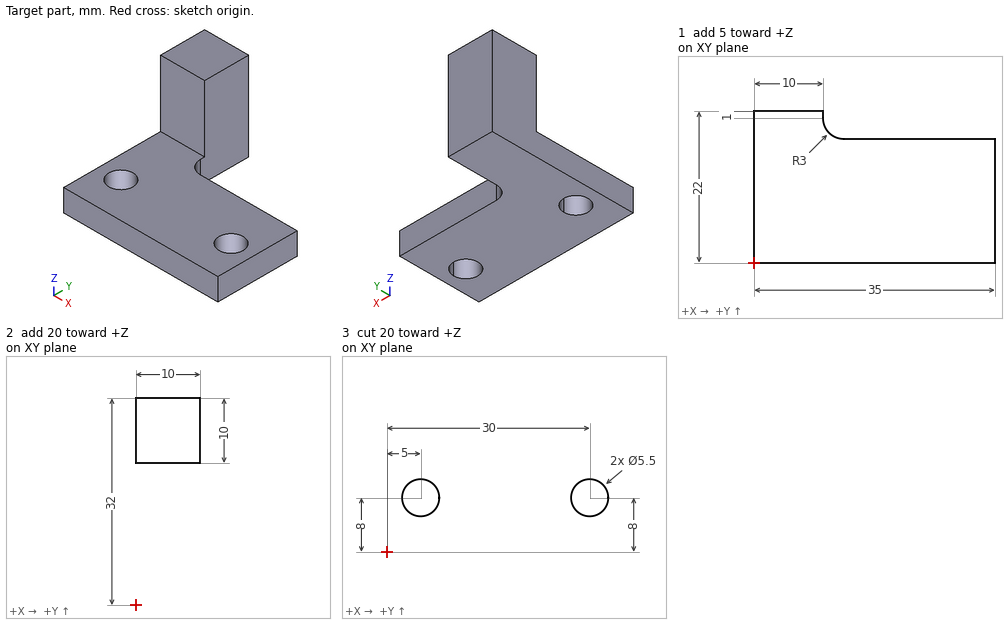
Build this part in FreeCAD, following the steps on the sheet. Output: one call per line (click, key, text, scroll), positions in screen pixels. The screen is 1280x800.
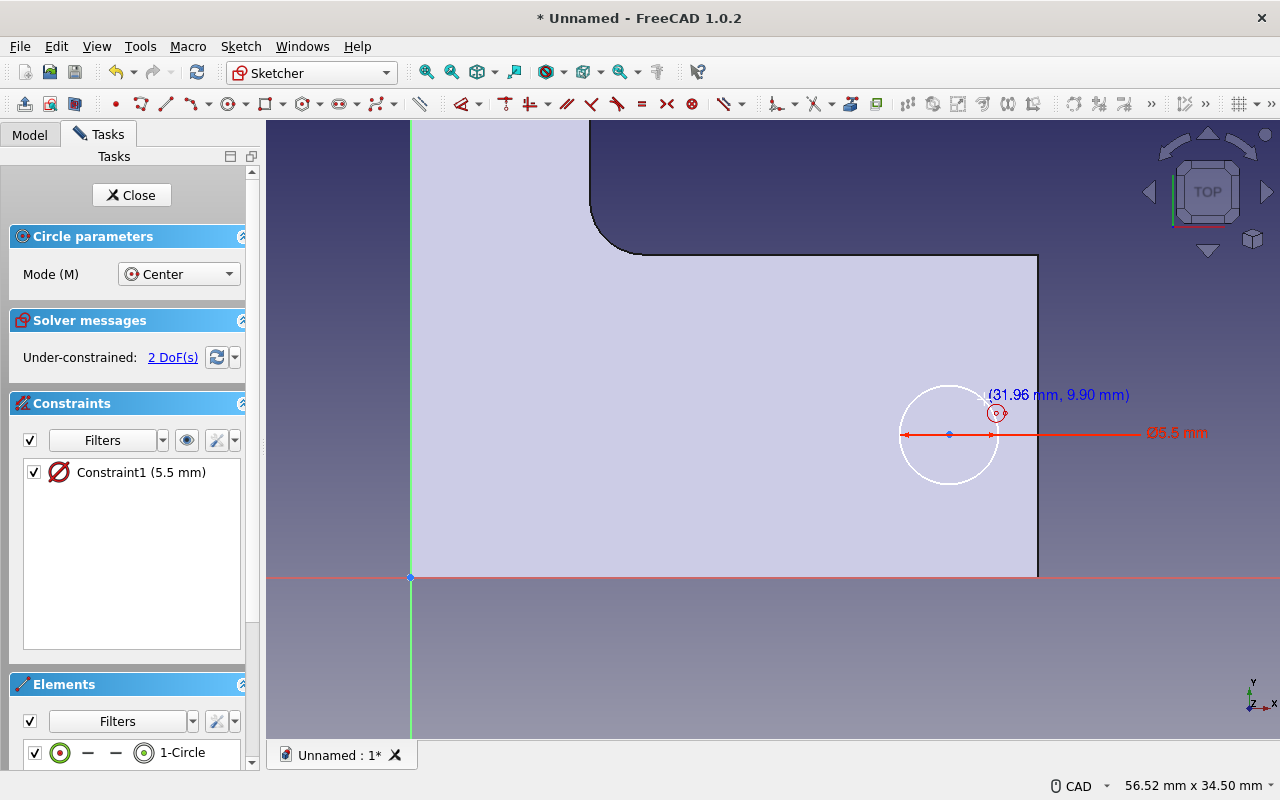
click(500, 434)
move(535, 399)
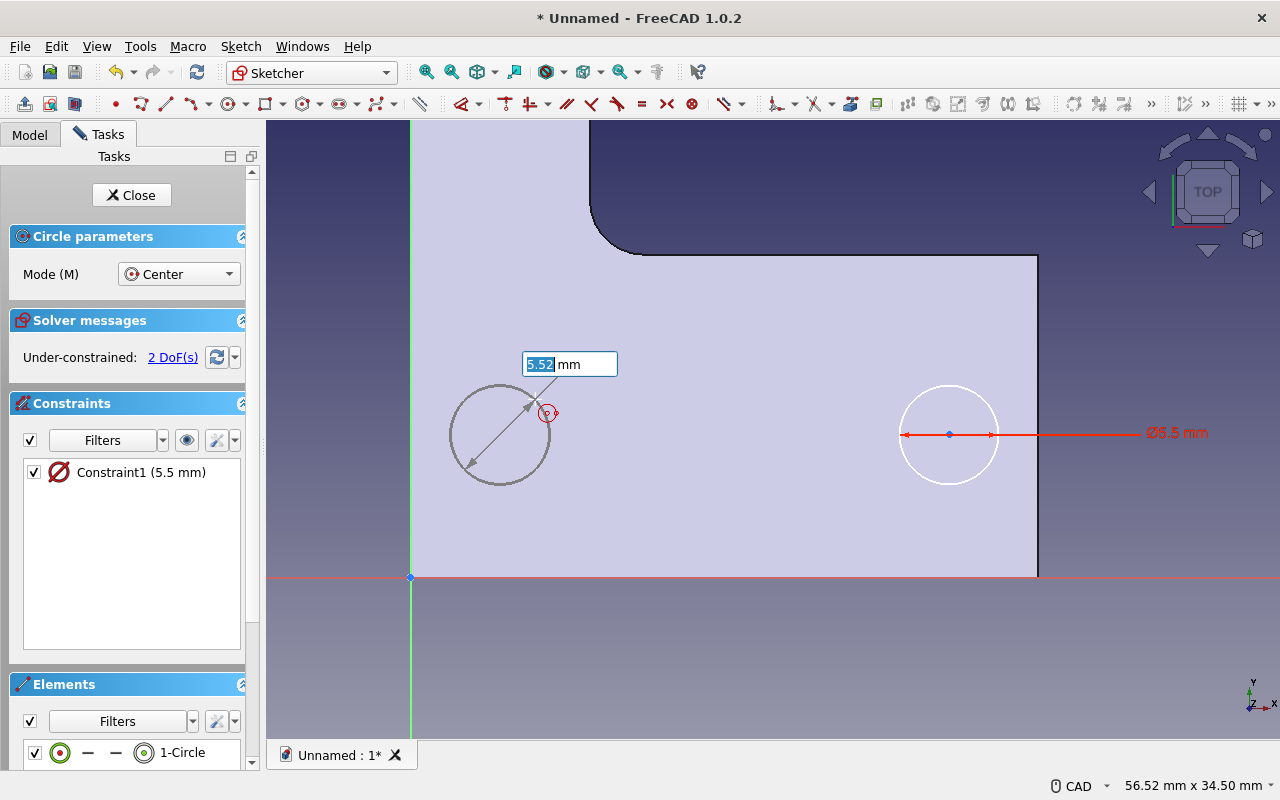
text(5.5)
key(Return)
key(Escape)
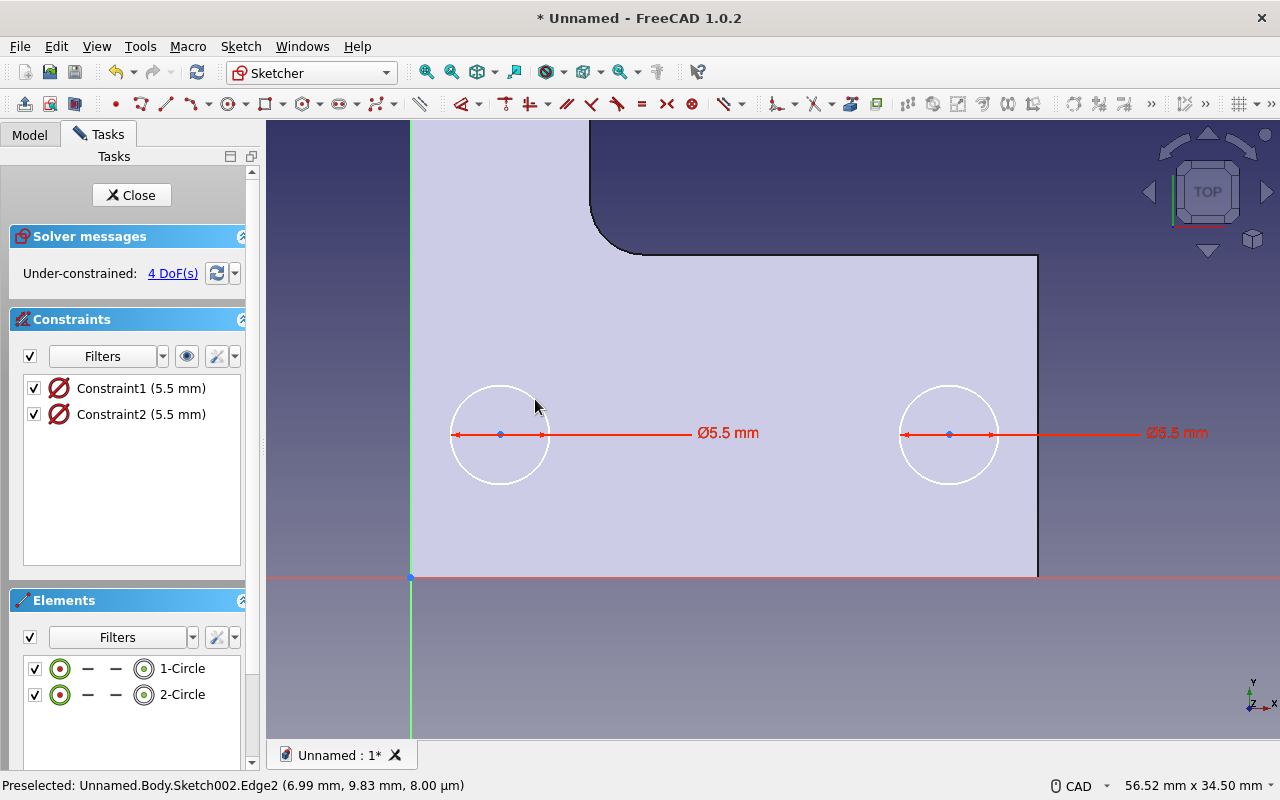
key(d)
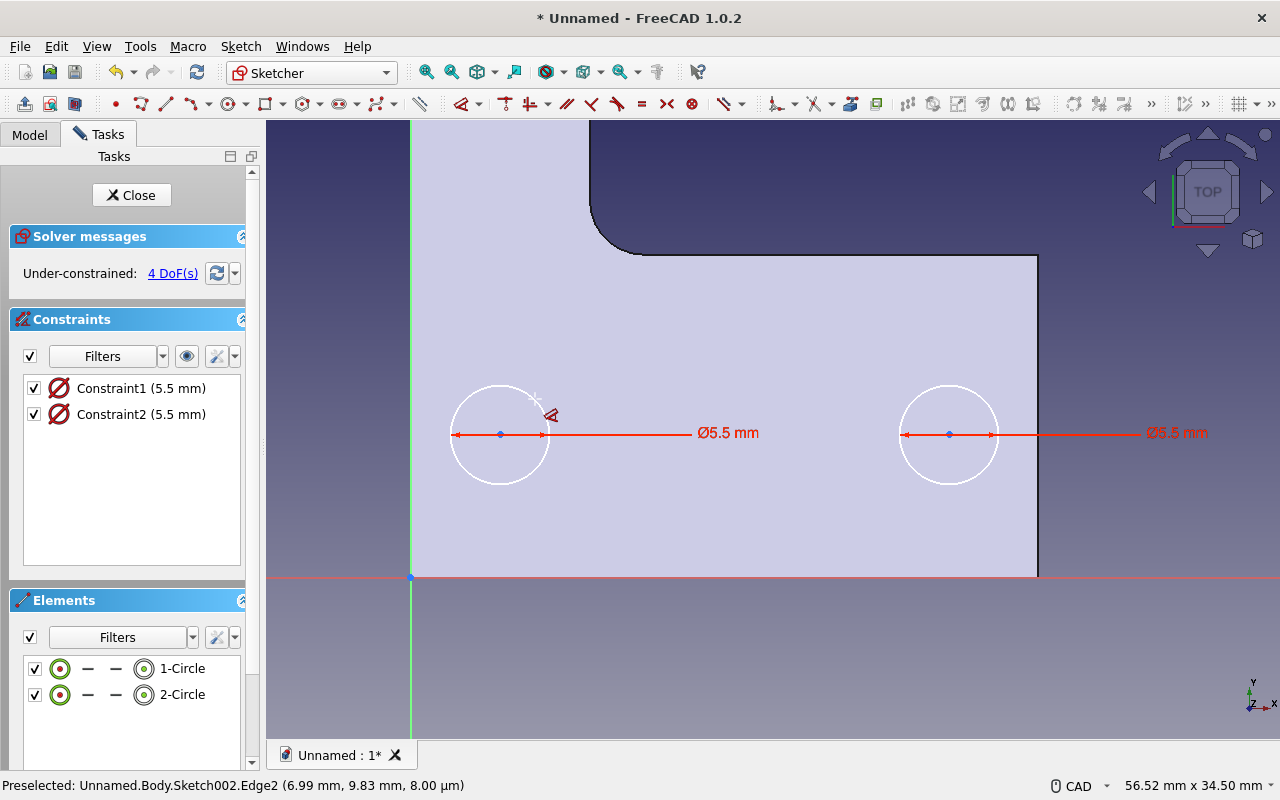
click(949, 435)
click(377, 506)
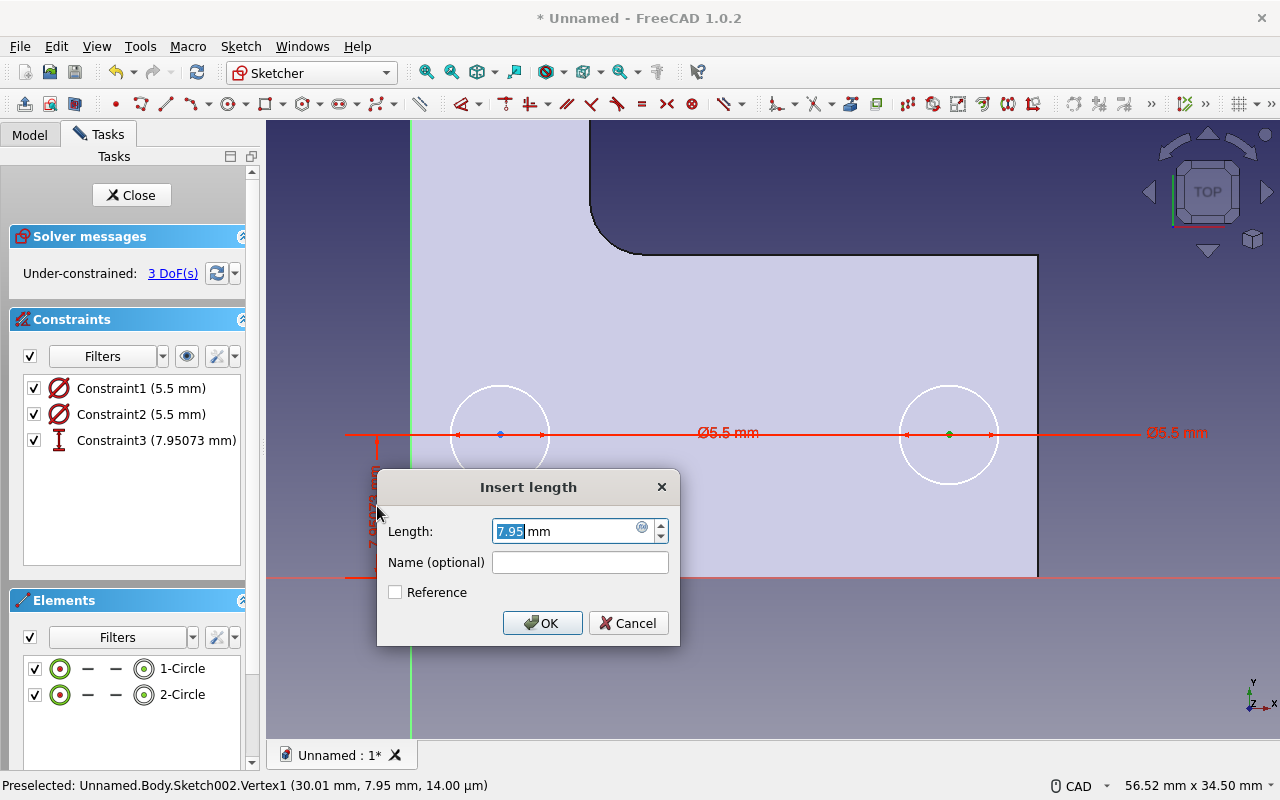
text(8)
key(Return)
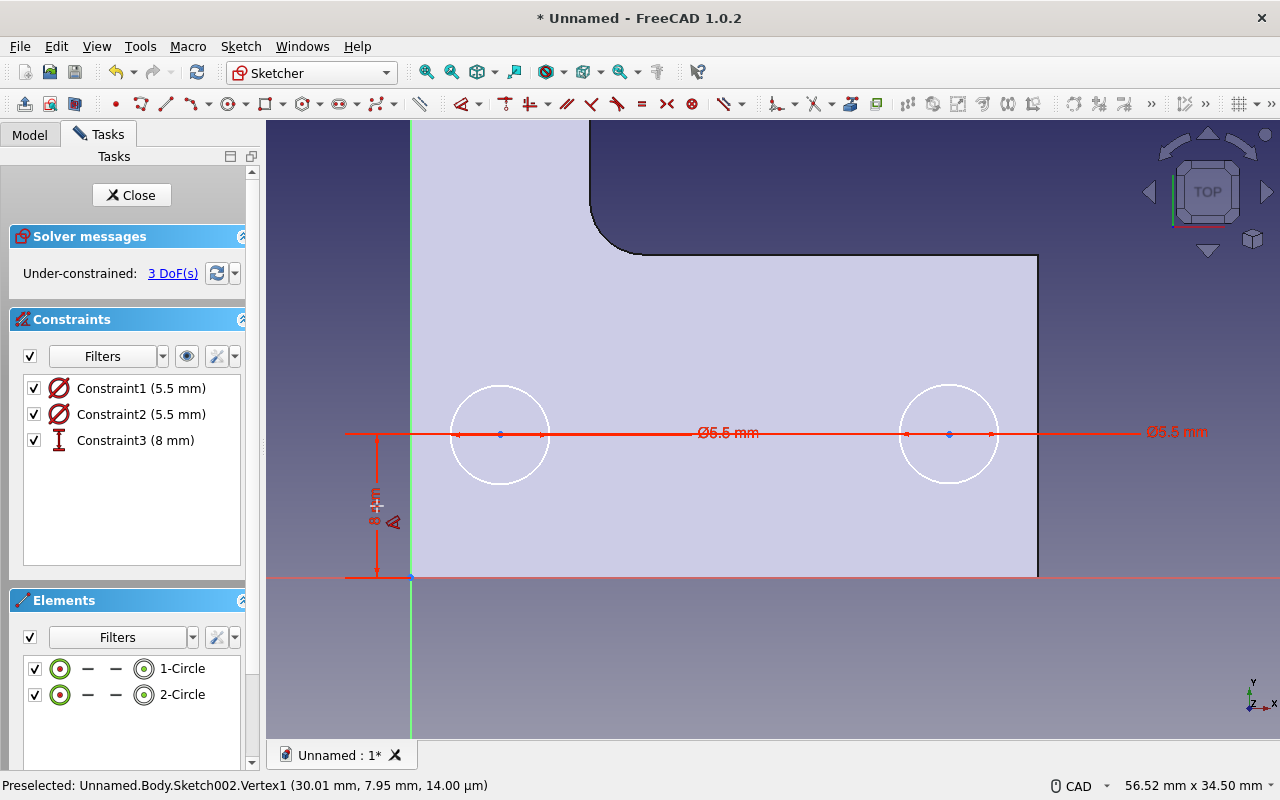
click(500, 435)
click(455, 612)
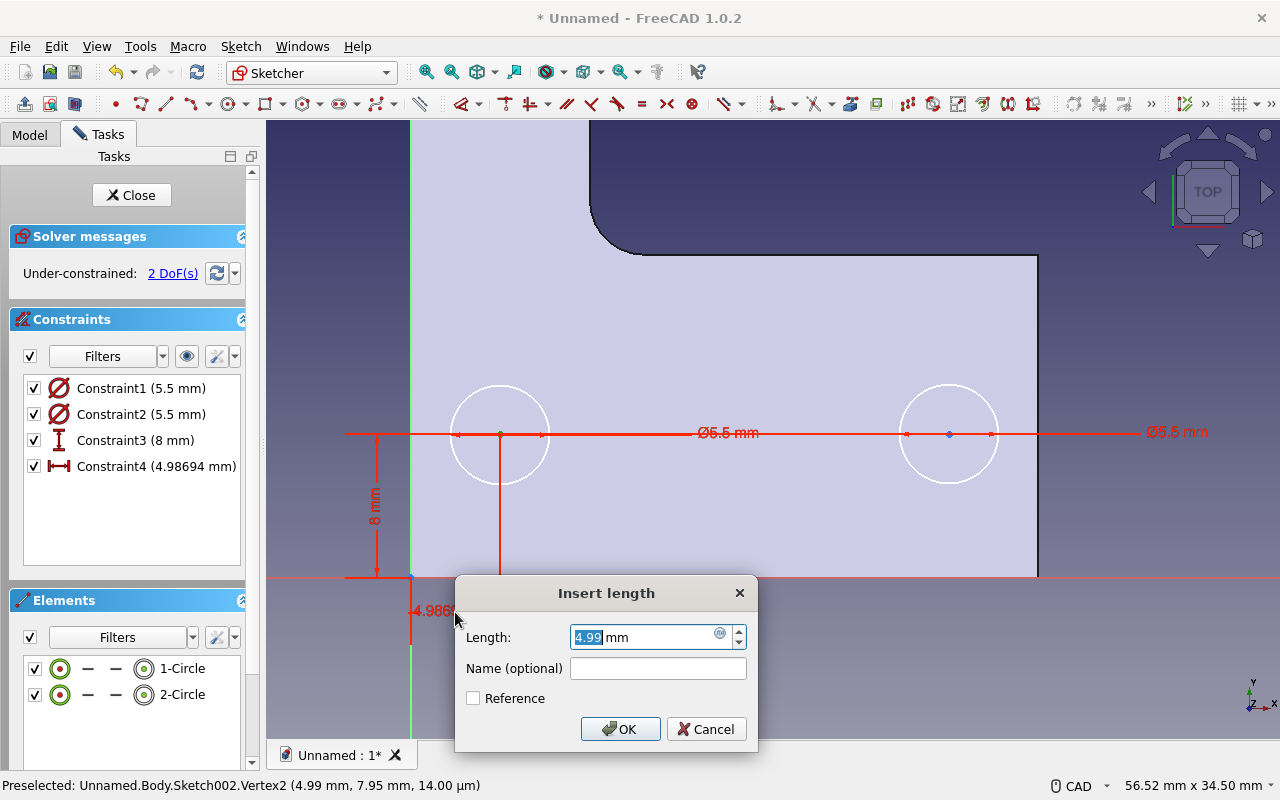
text(5)
key(Return)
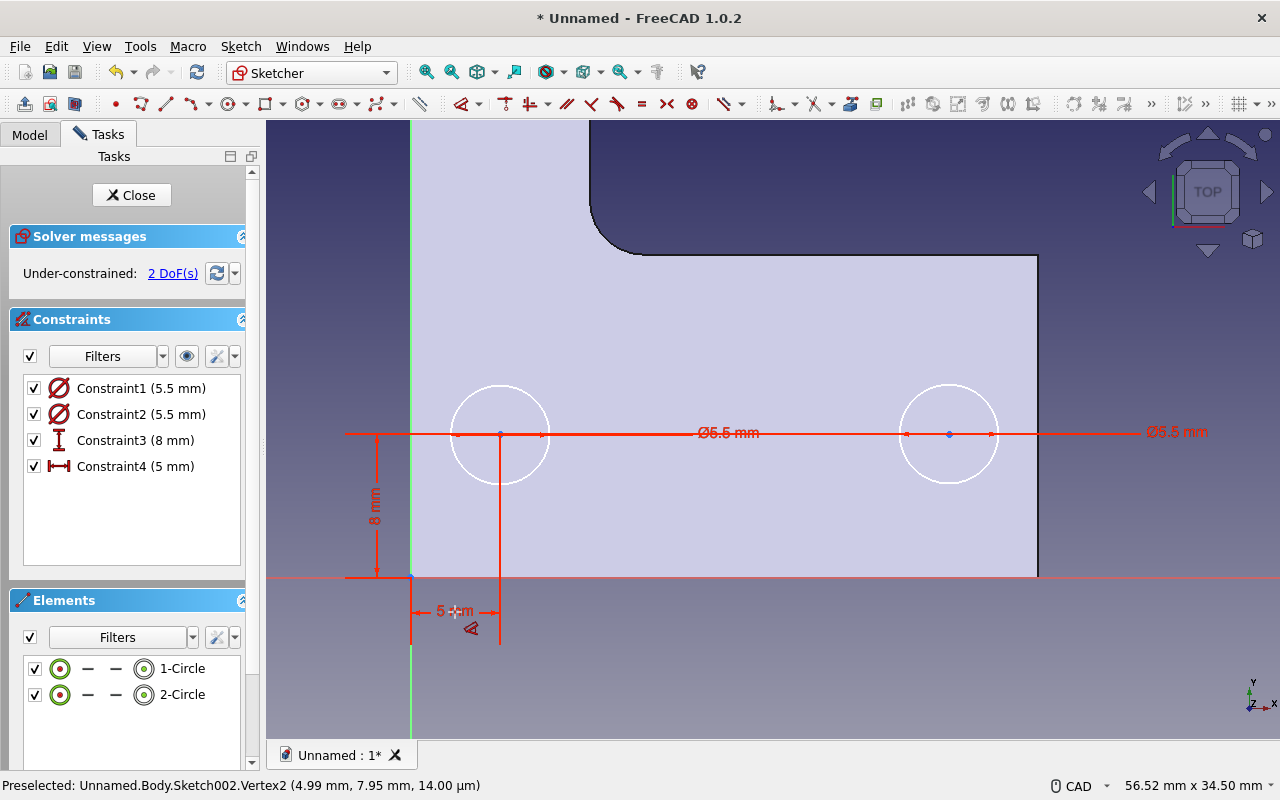
click(500, 435)
click(377, 474)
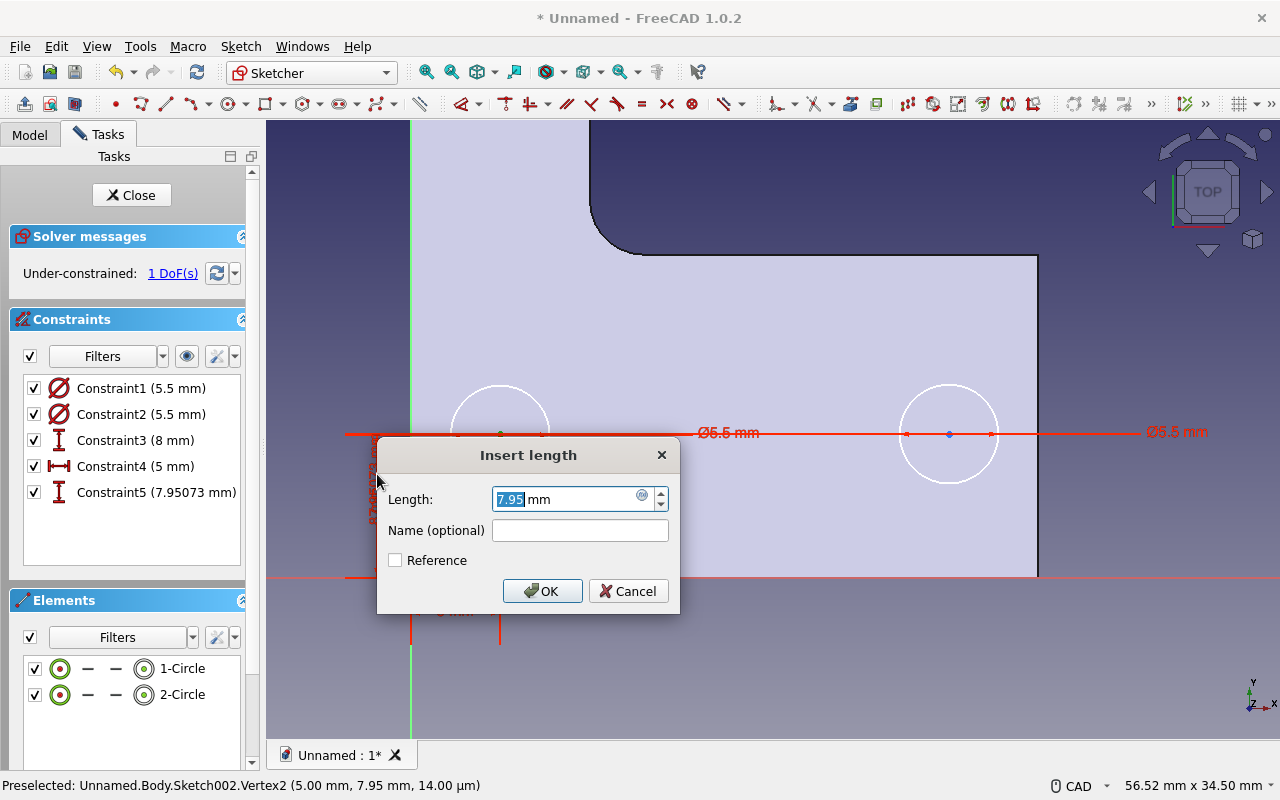
text(8)
key(Return)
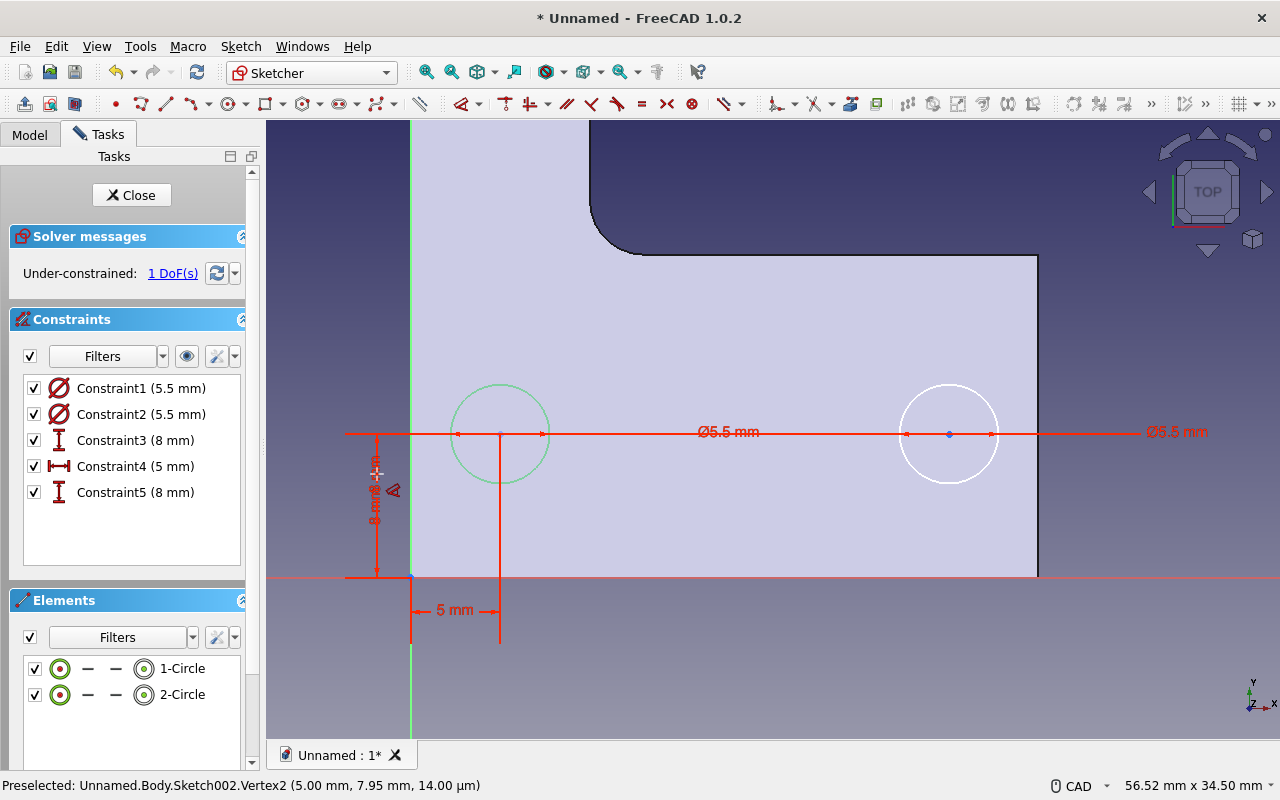
click(949, 434)
click(680, 612)